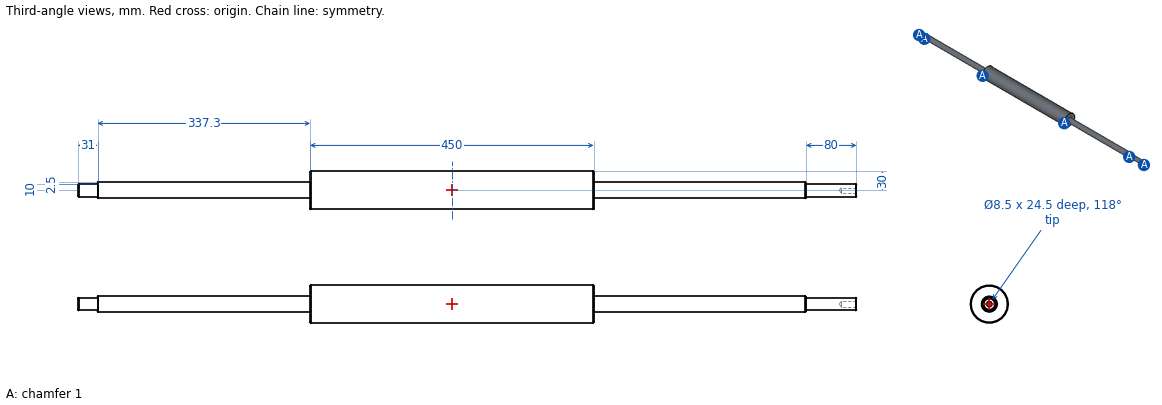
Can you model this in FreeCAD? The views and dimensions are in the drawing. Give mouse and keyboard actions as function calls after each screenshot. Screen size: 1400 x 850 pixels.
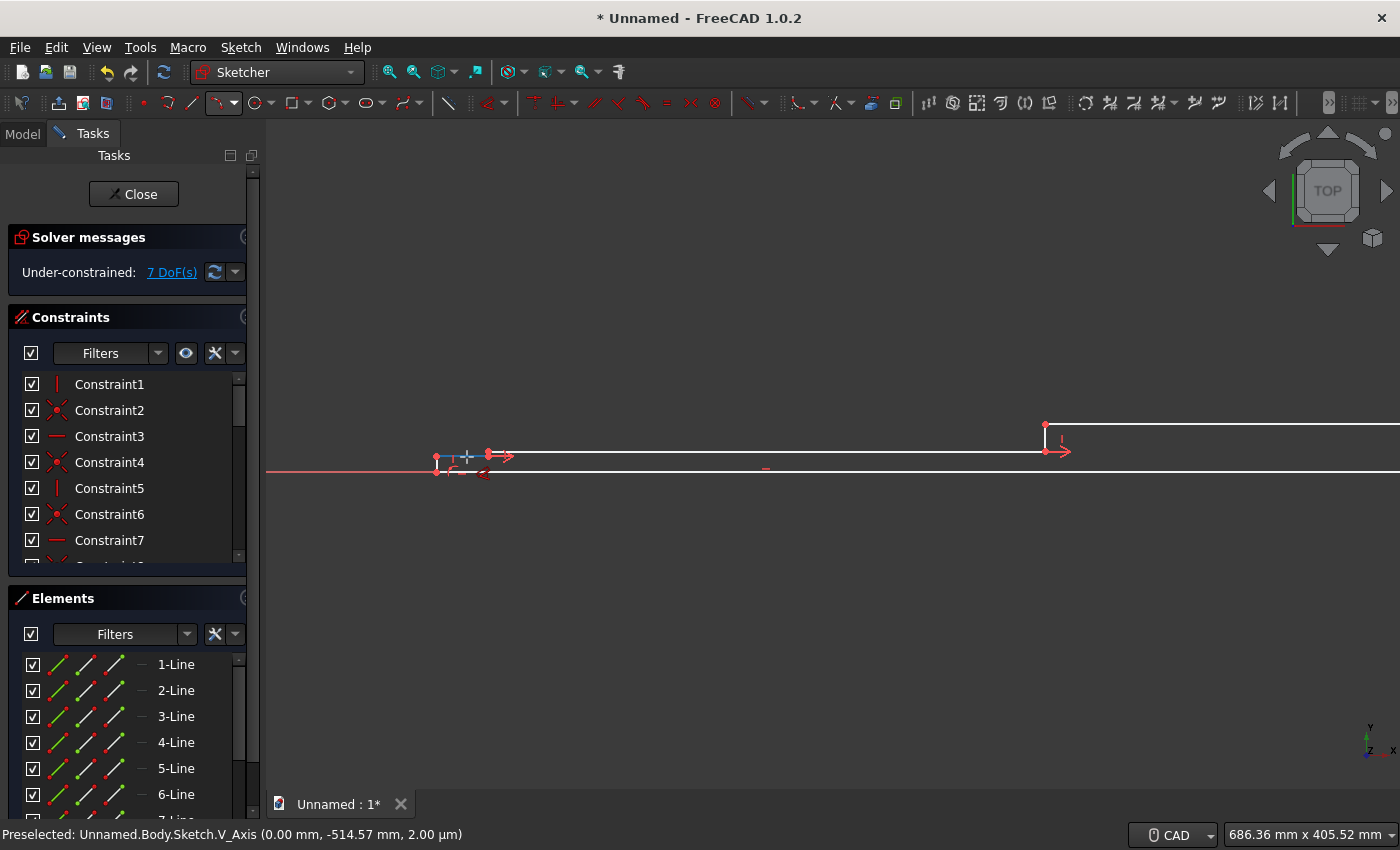
click(468, 456)
click(463, 490)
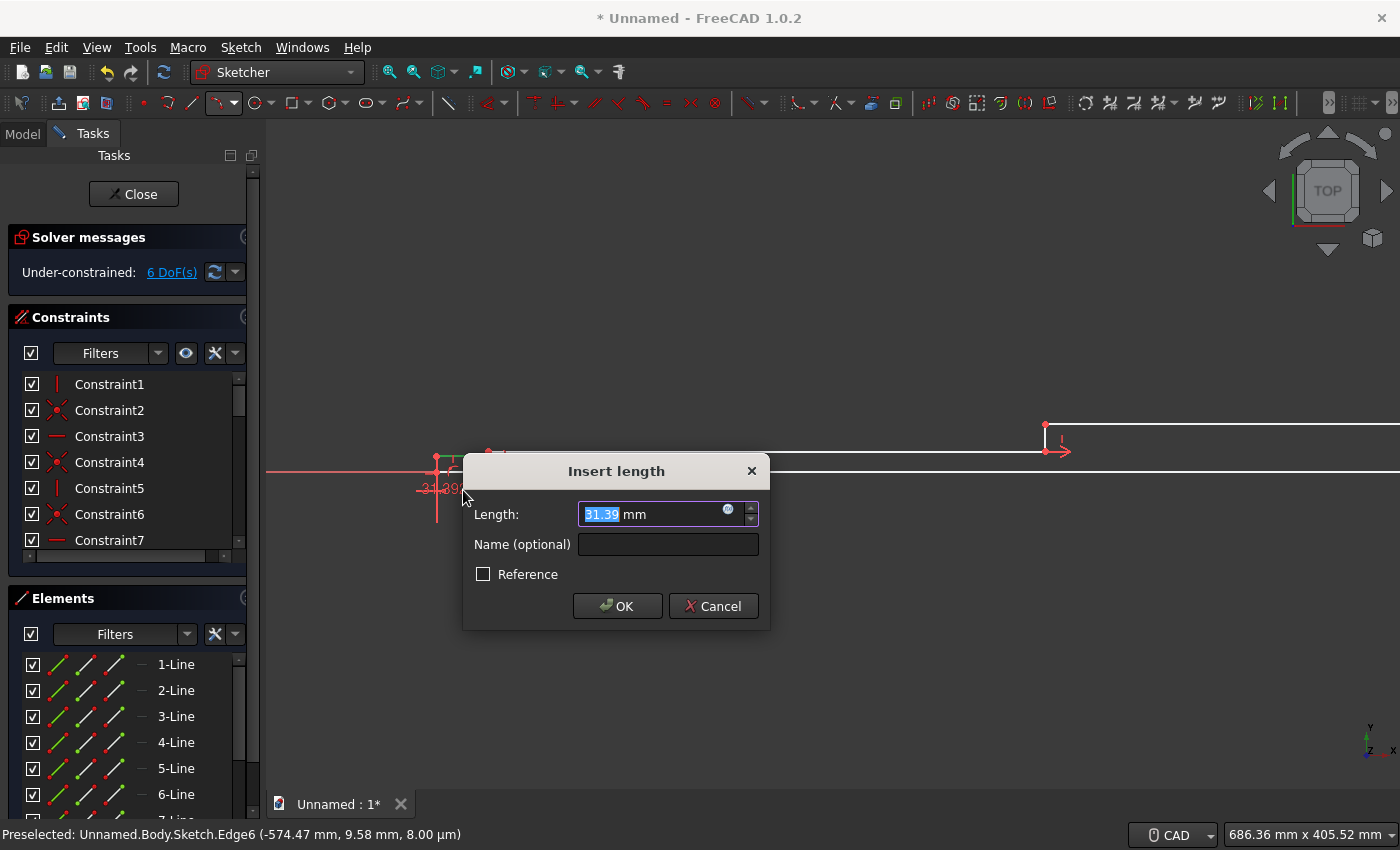
text(31)
key(Return)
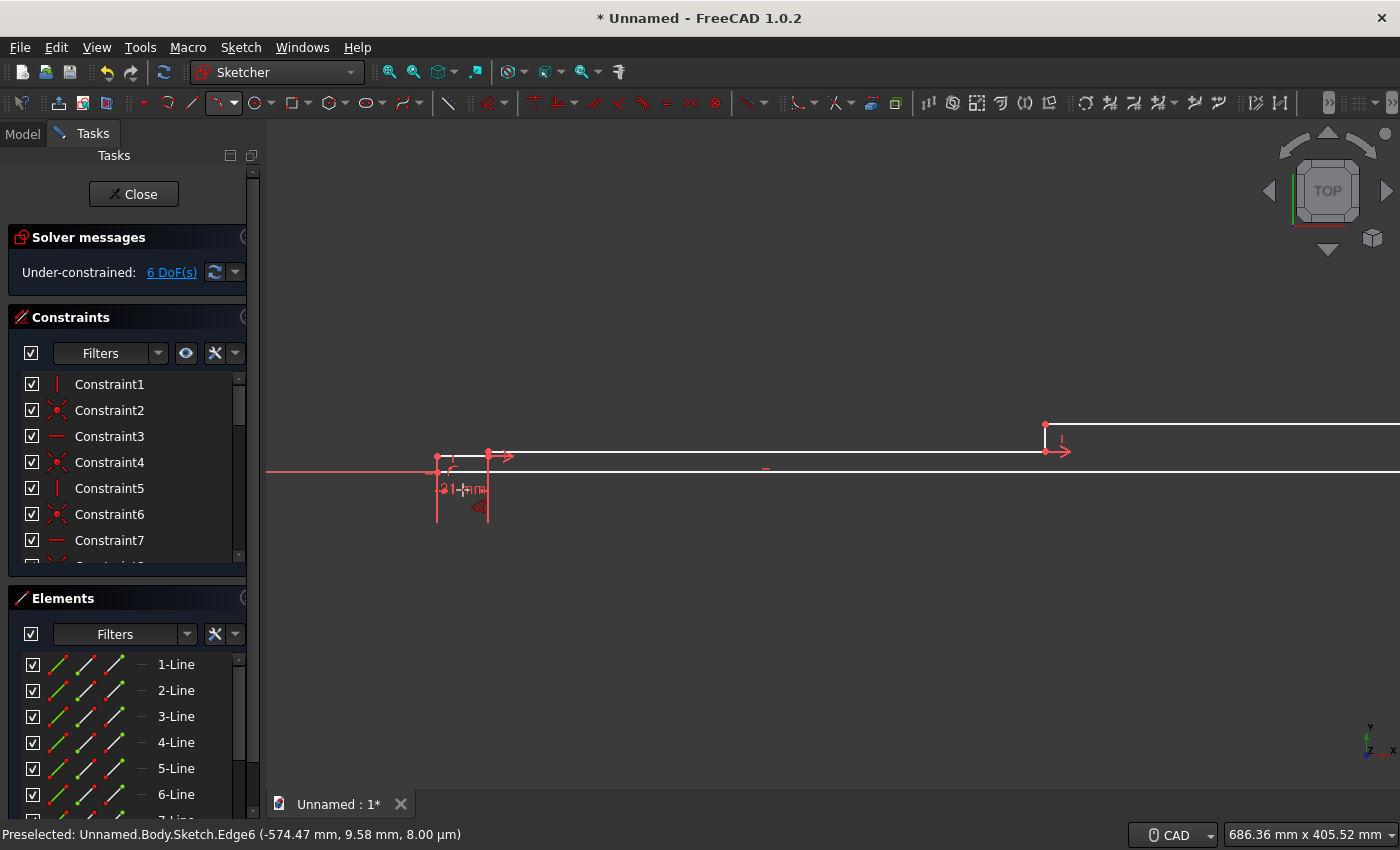
scroll(437, 464, up, 5)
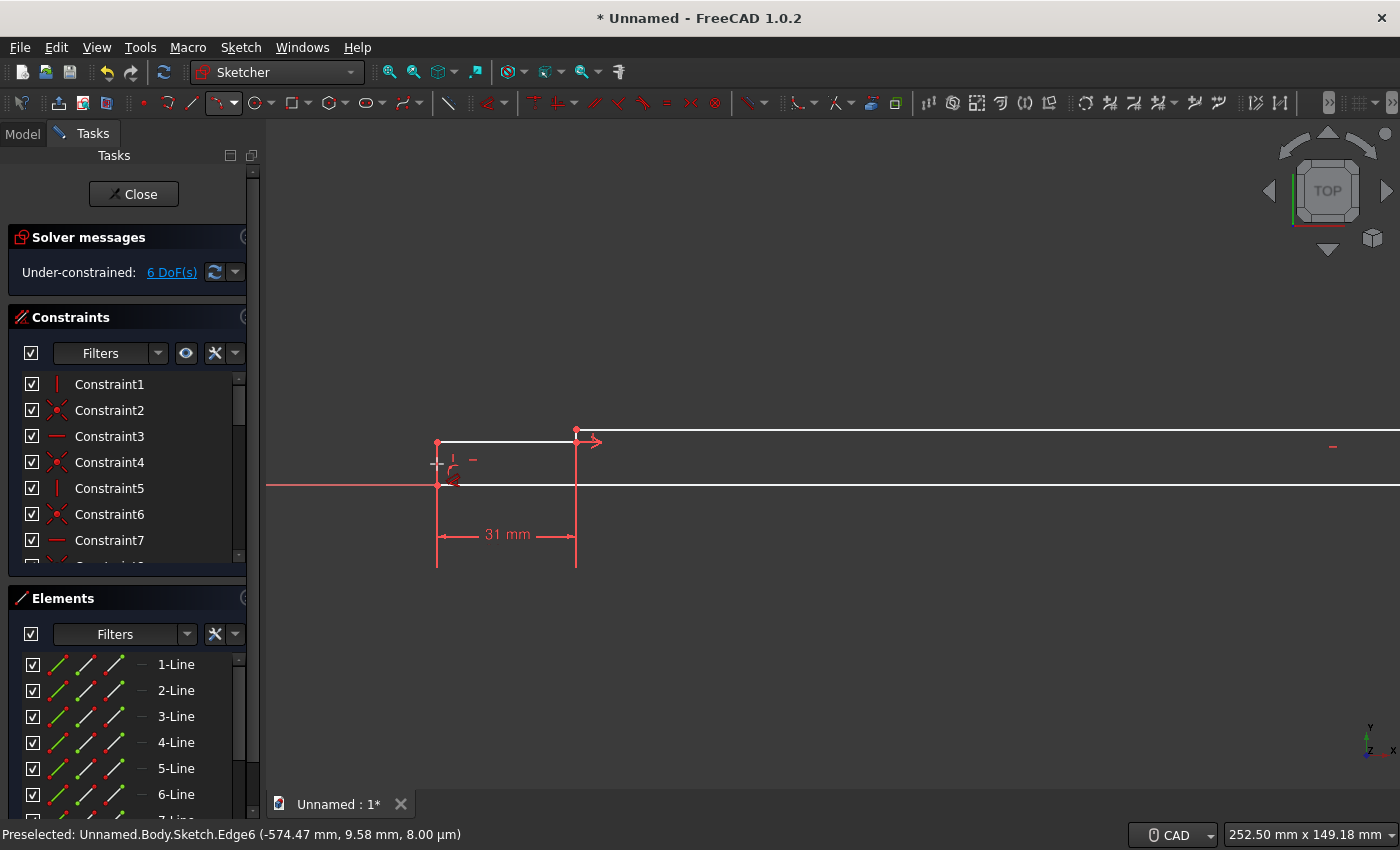
click(437, 464)
click(403, 464)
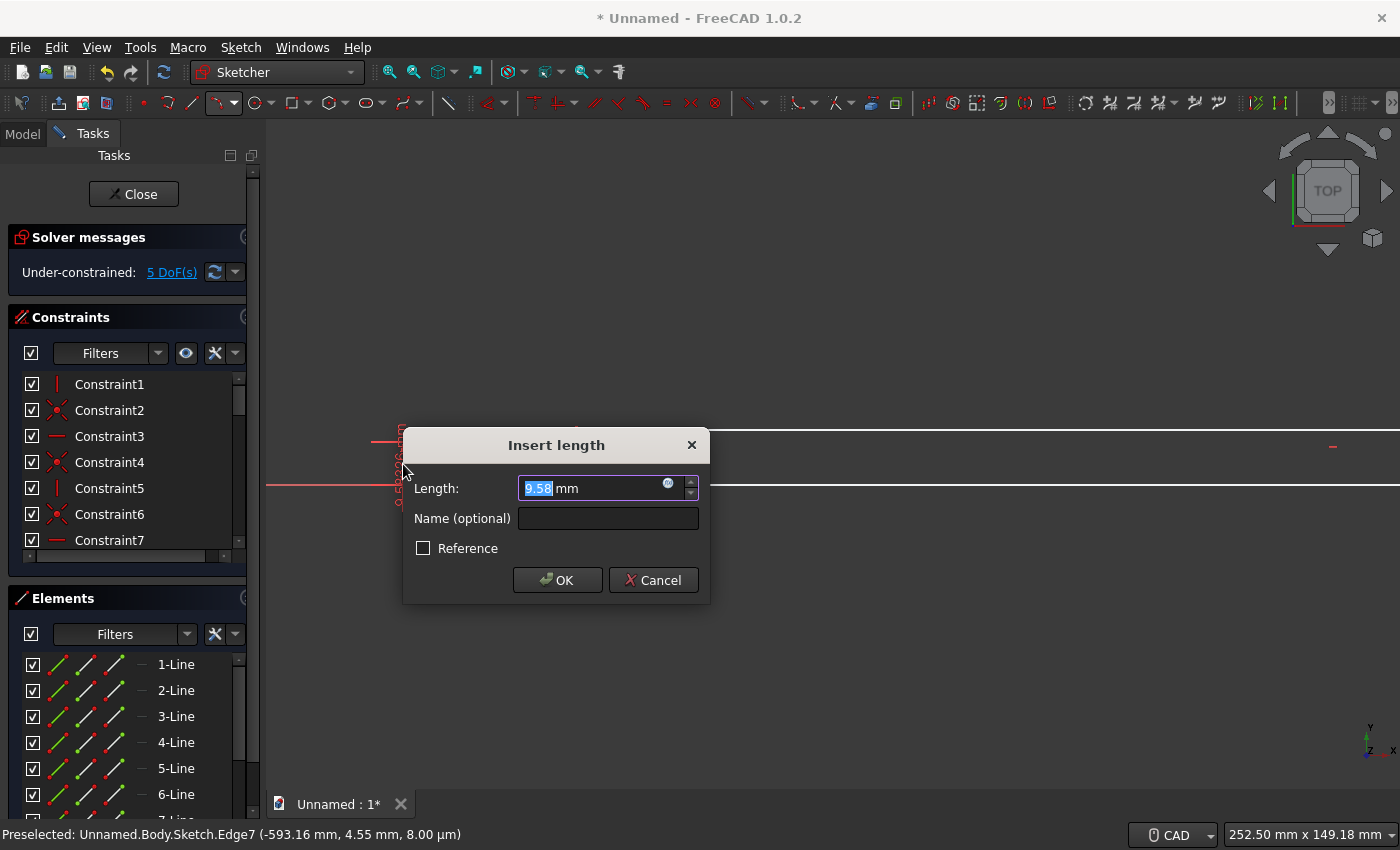
text(10)
key(Return)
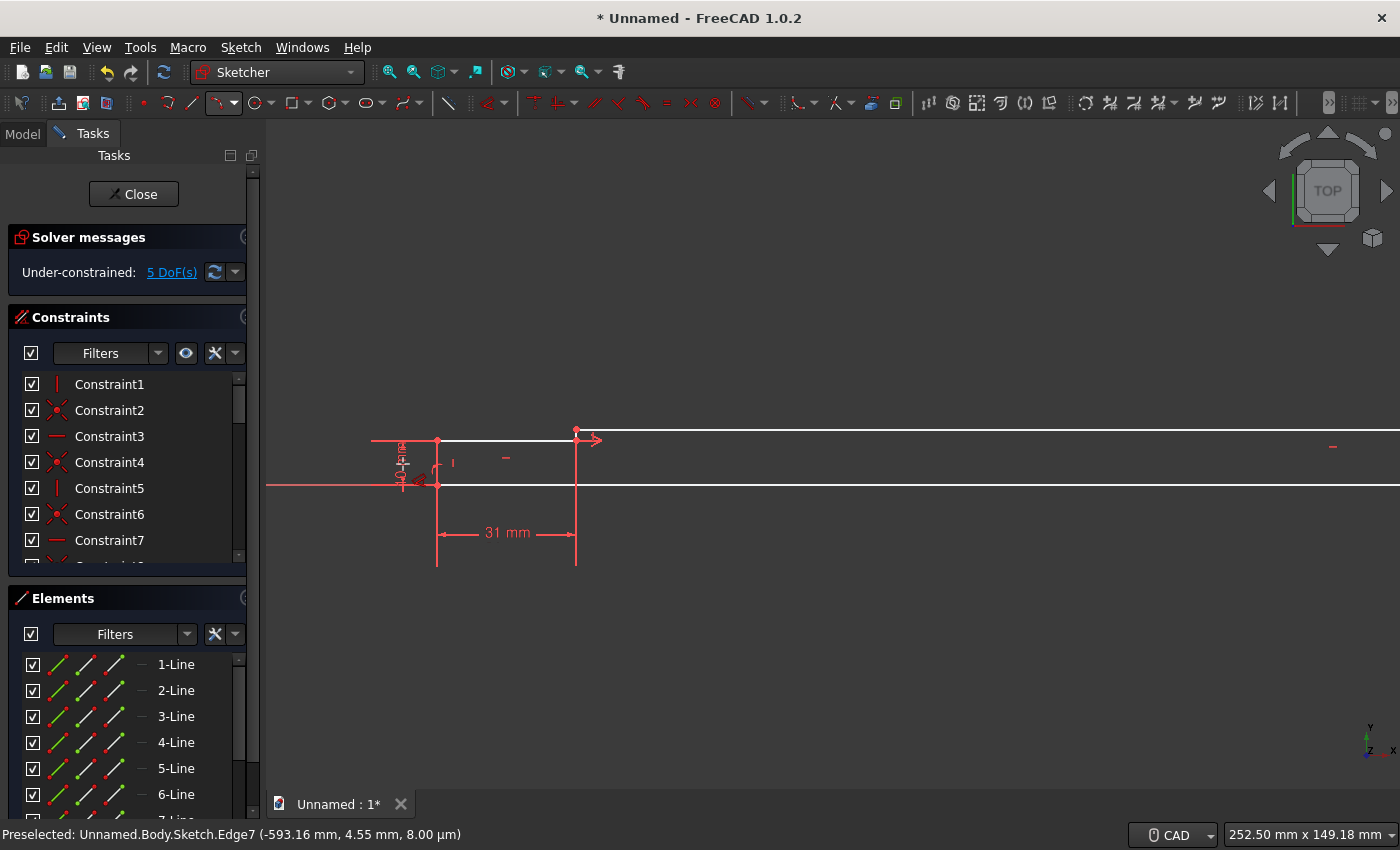
scroll(460, 458, down, 11)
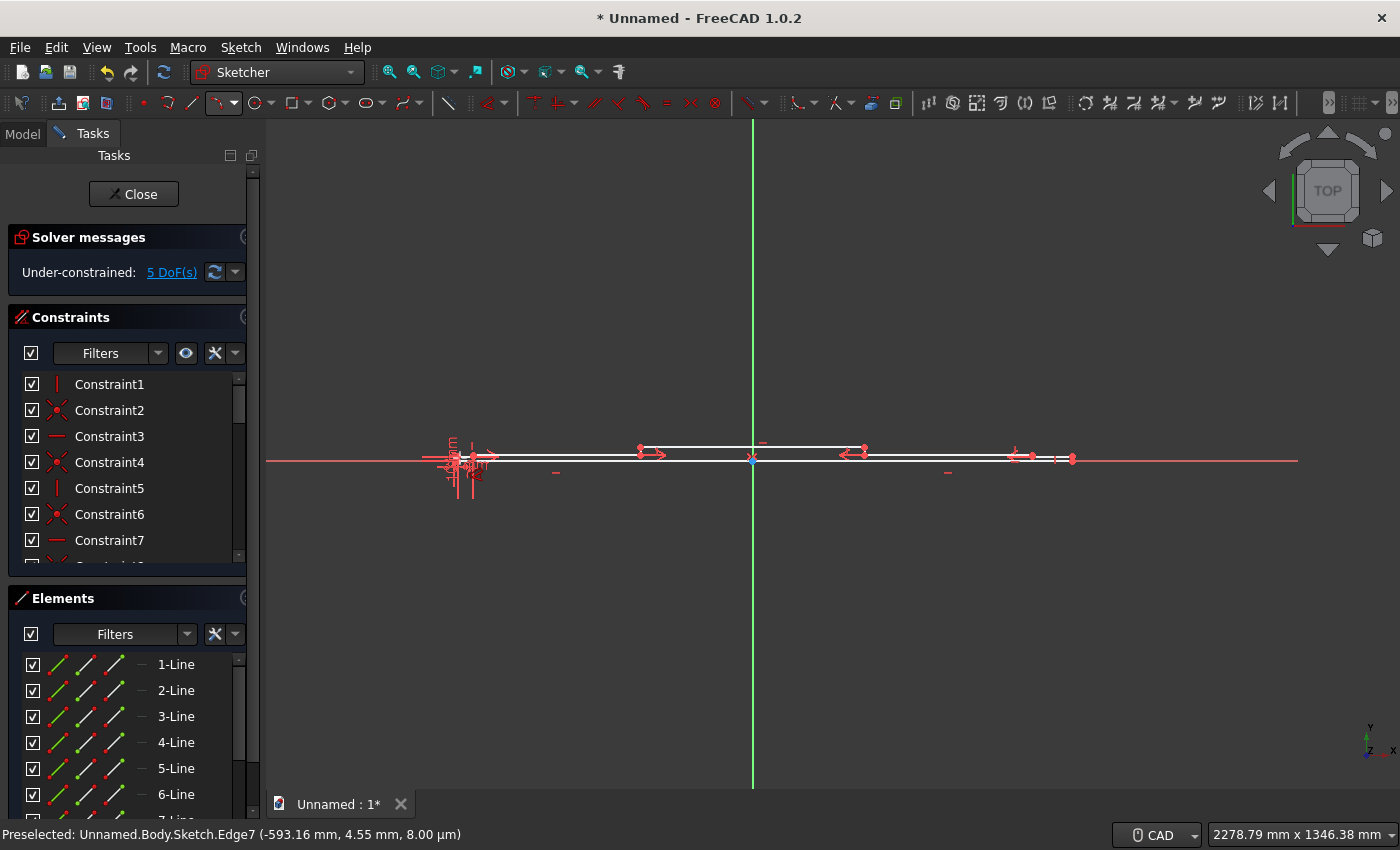
scroll(1061, 457, up, 6)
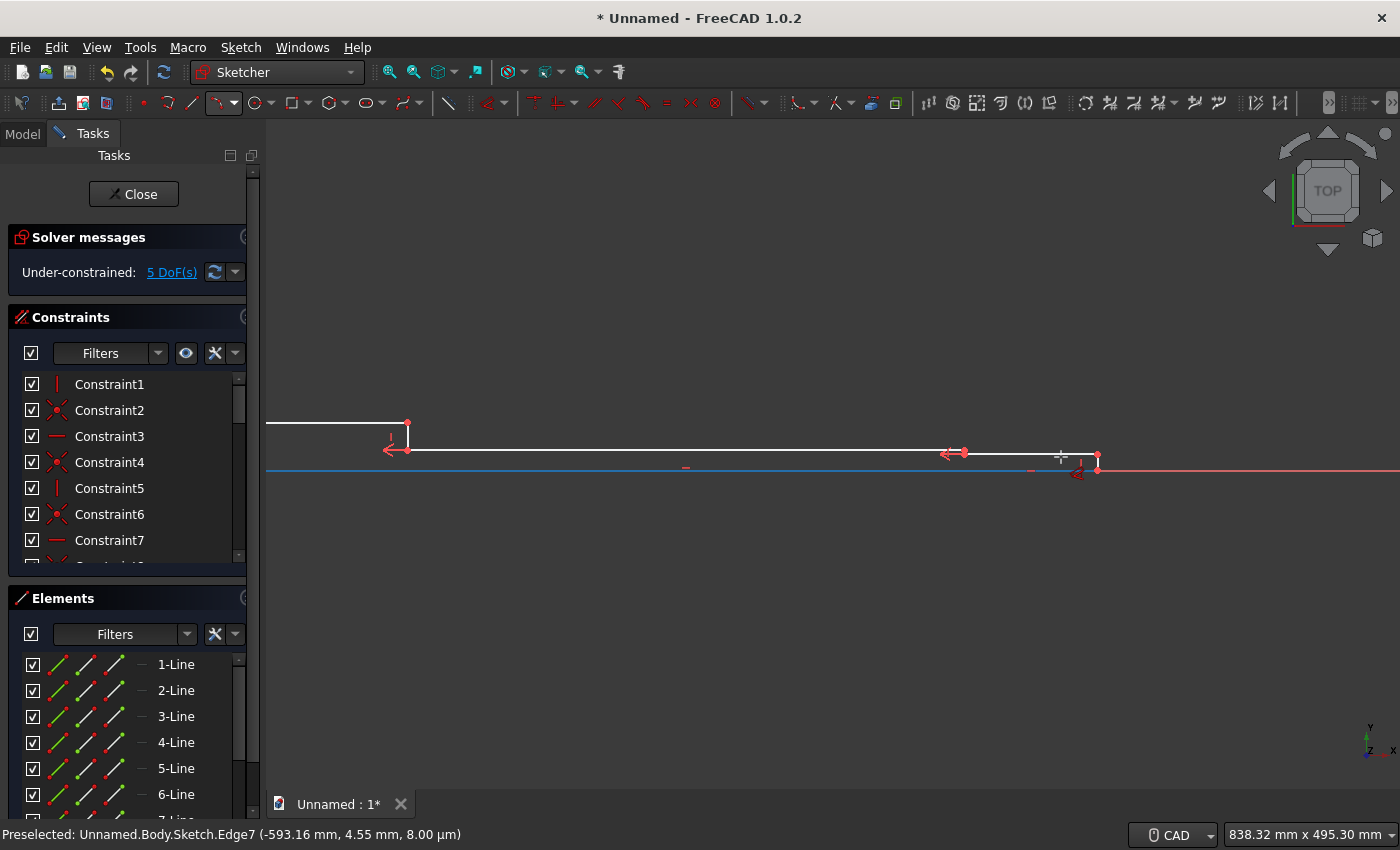
click(1058, 454)
click(1031, 488)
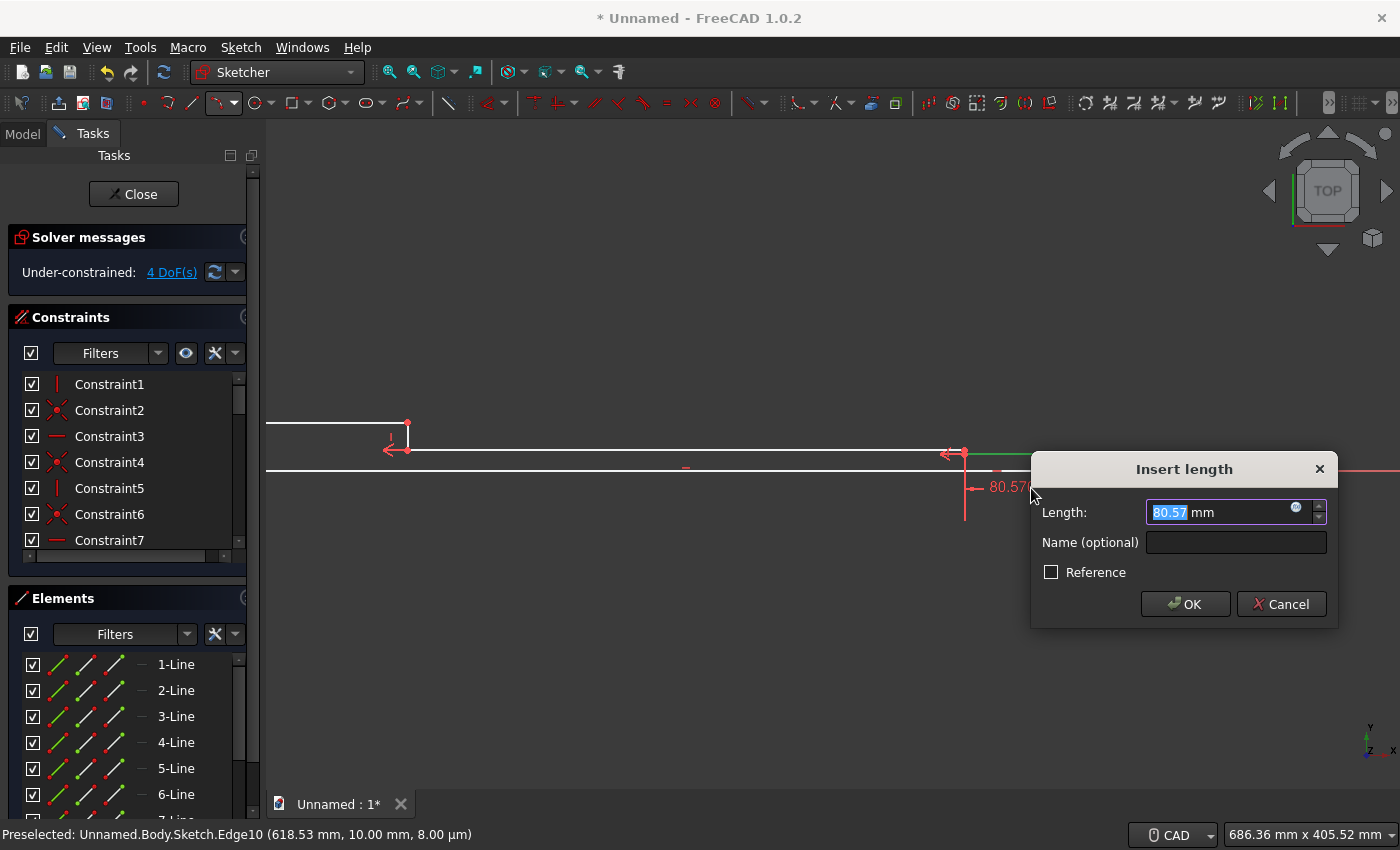
text(80)
key(Return)